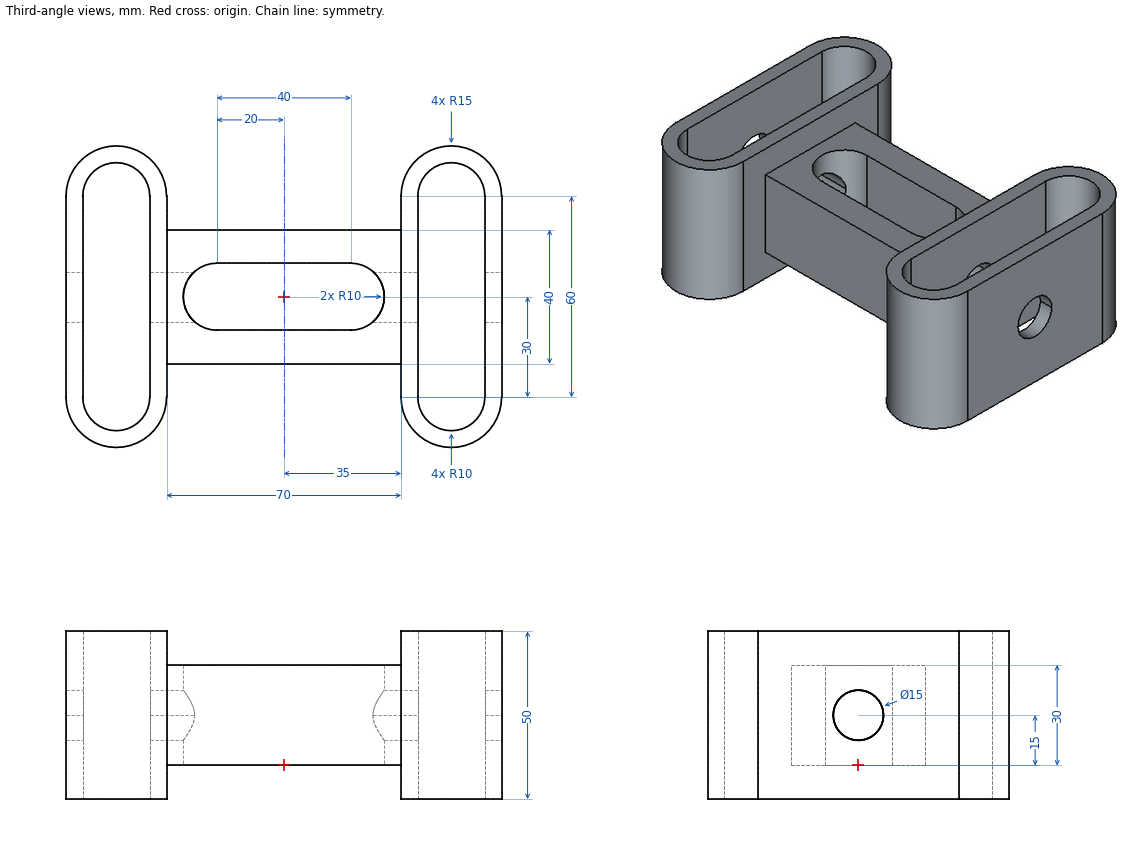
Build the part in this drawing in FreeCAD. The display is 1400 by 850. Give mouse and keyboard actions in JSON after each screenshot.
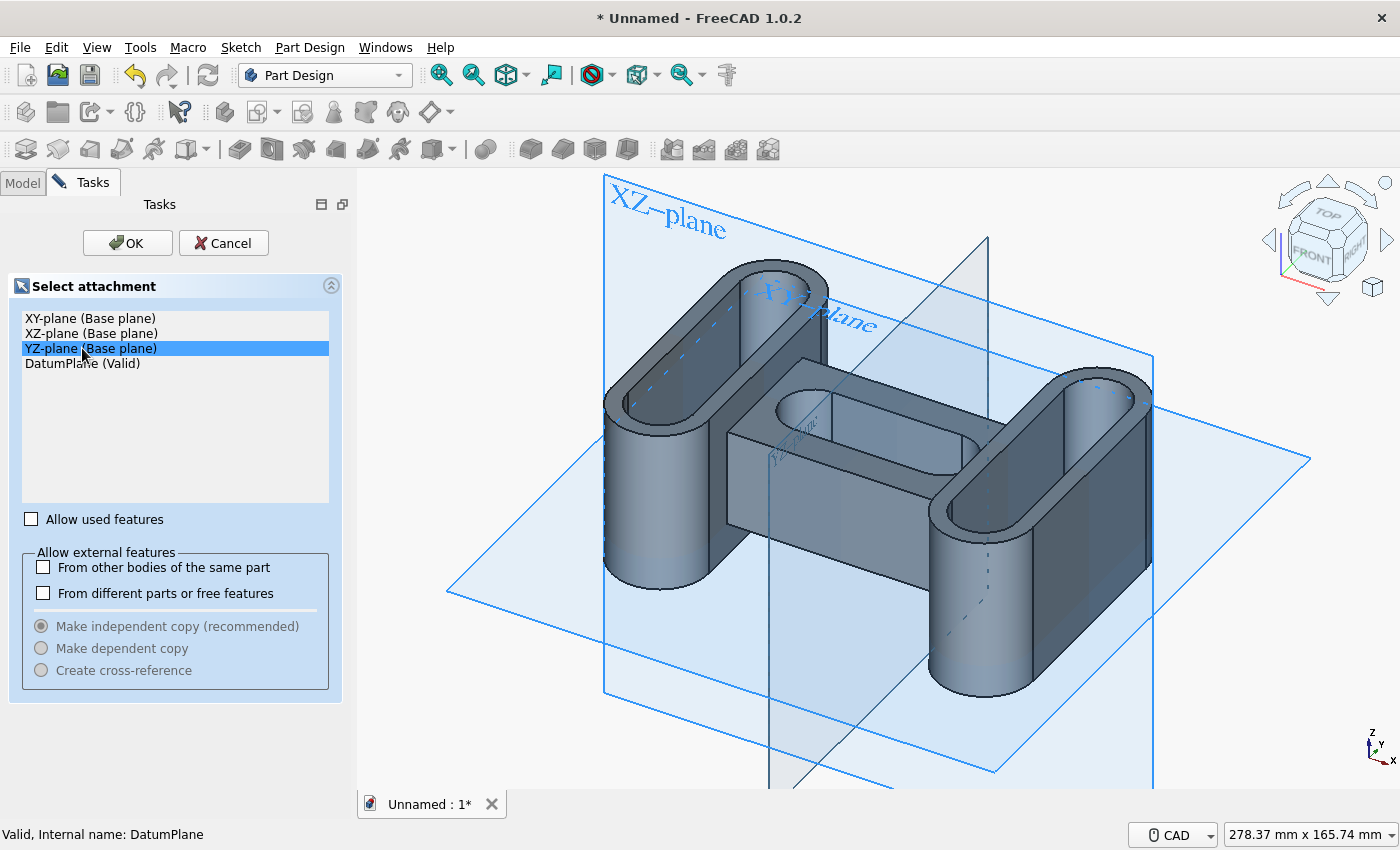
{"action": "left_click", "coordinate": [128, 243]}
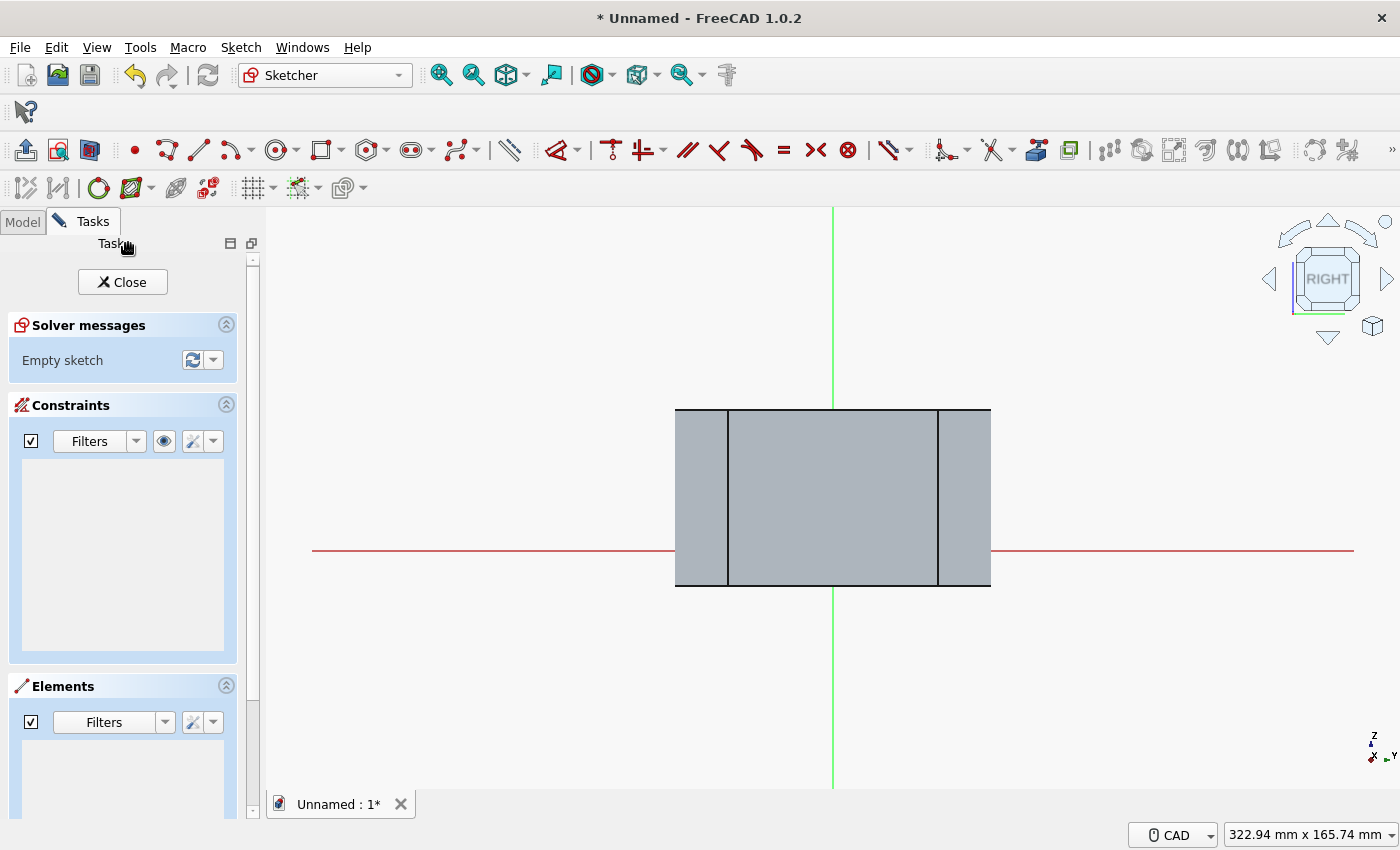
{"action": "key", "text": "q s"}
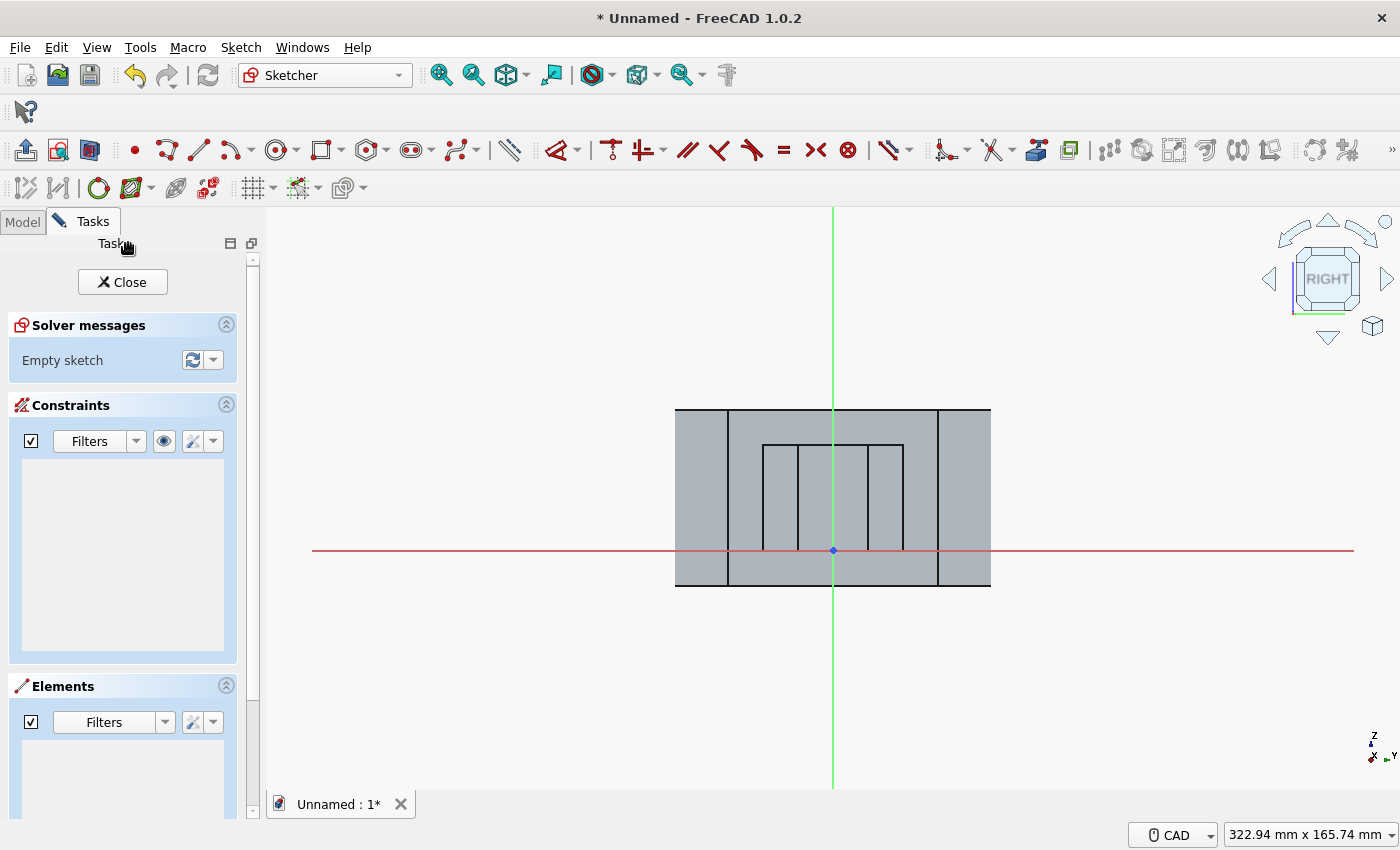
{"action": "scroll", "coordinate": [850, 514], "scroll_direction": "up", "scroll_amount": 8}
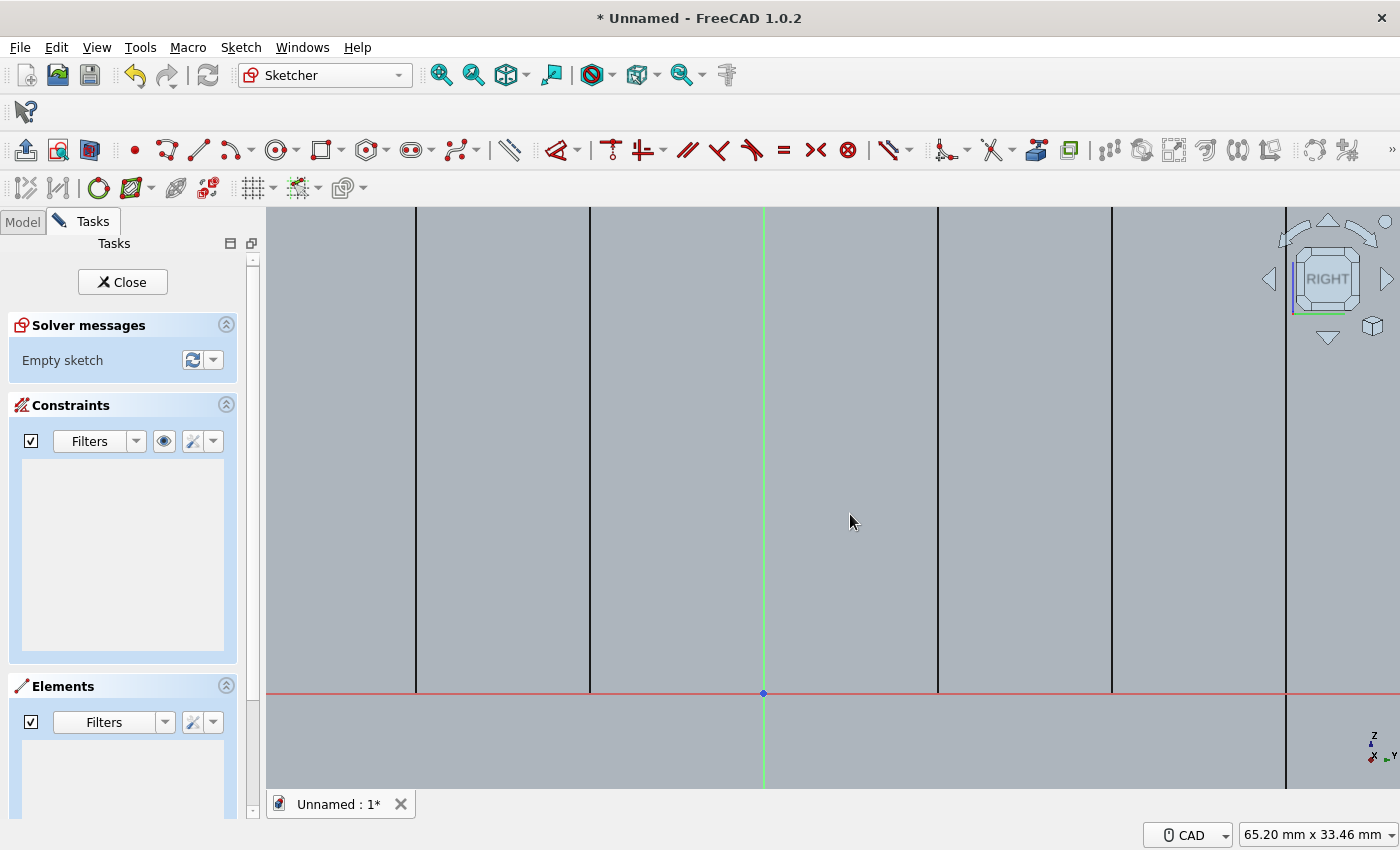
{"action": "left_click", "coordinate": [276, 150]}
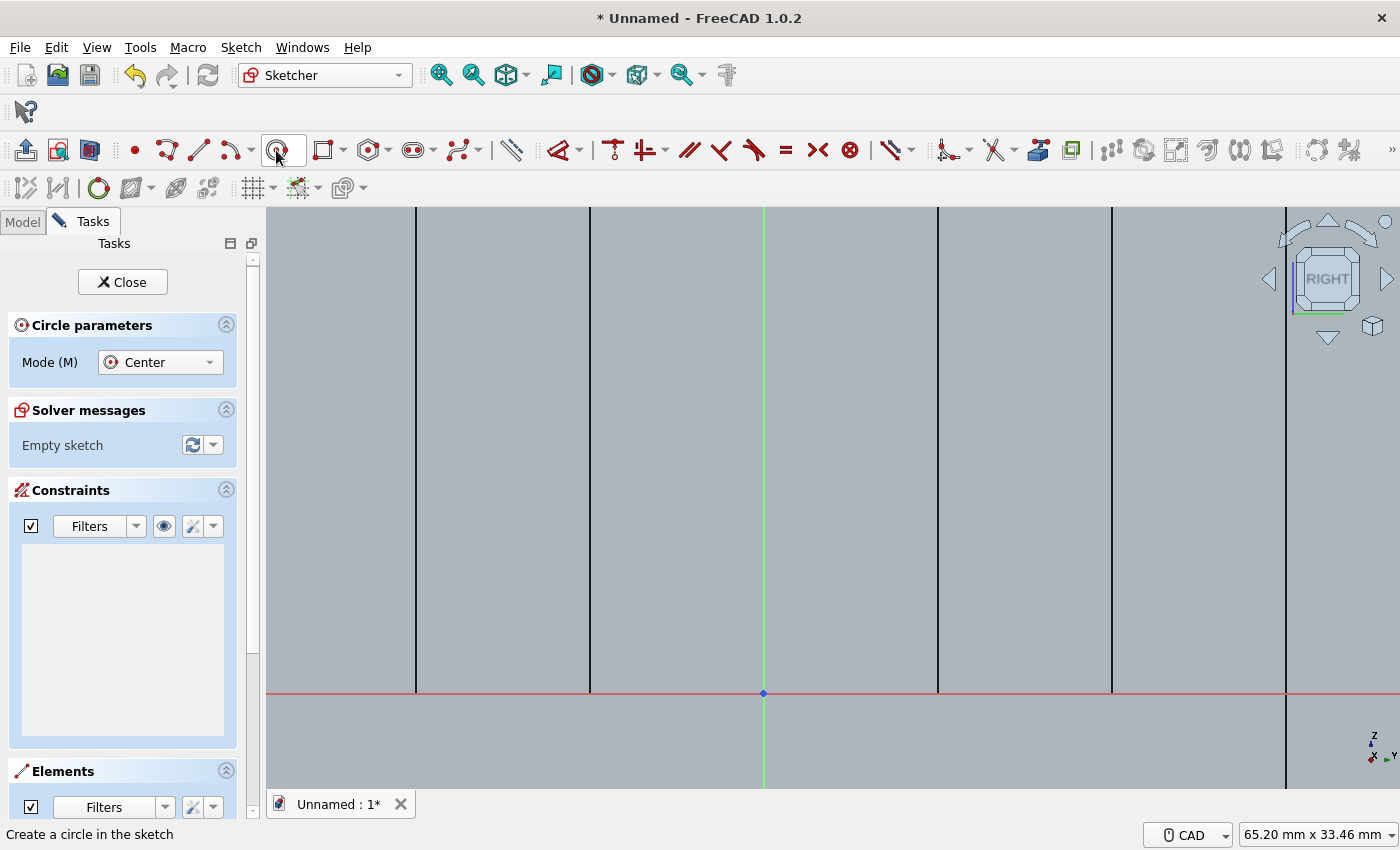
{"action": "left_click", "coordinate": [764, 433]}
{"action": "mouse_move", "coordinate": [856, 340]}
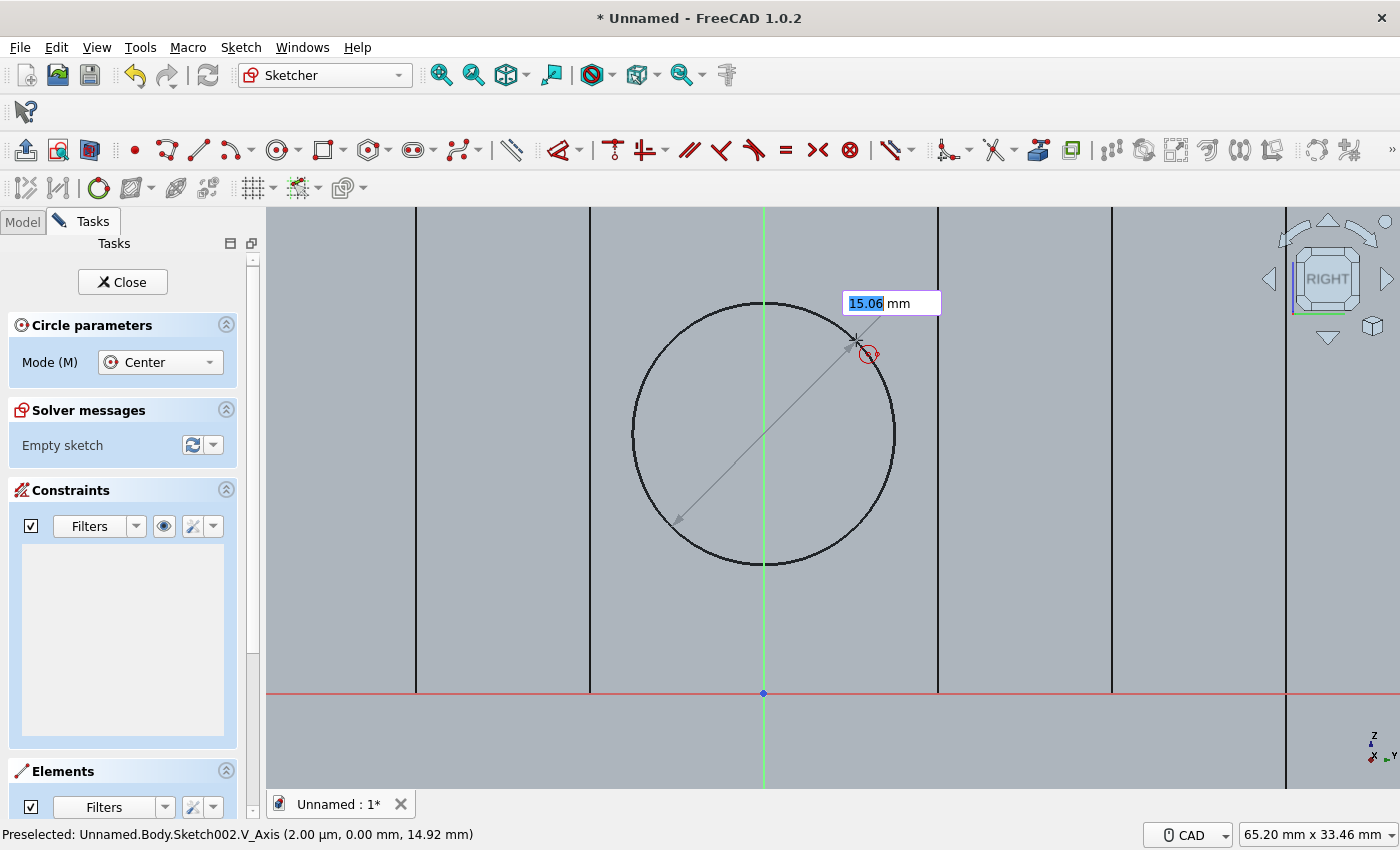
{"action": "type", "text": "15"}
{"action": "key", "text": "Return"}
{"action": "key", "text": "Escape"}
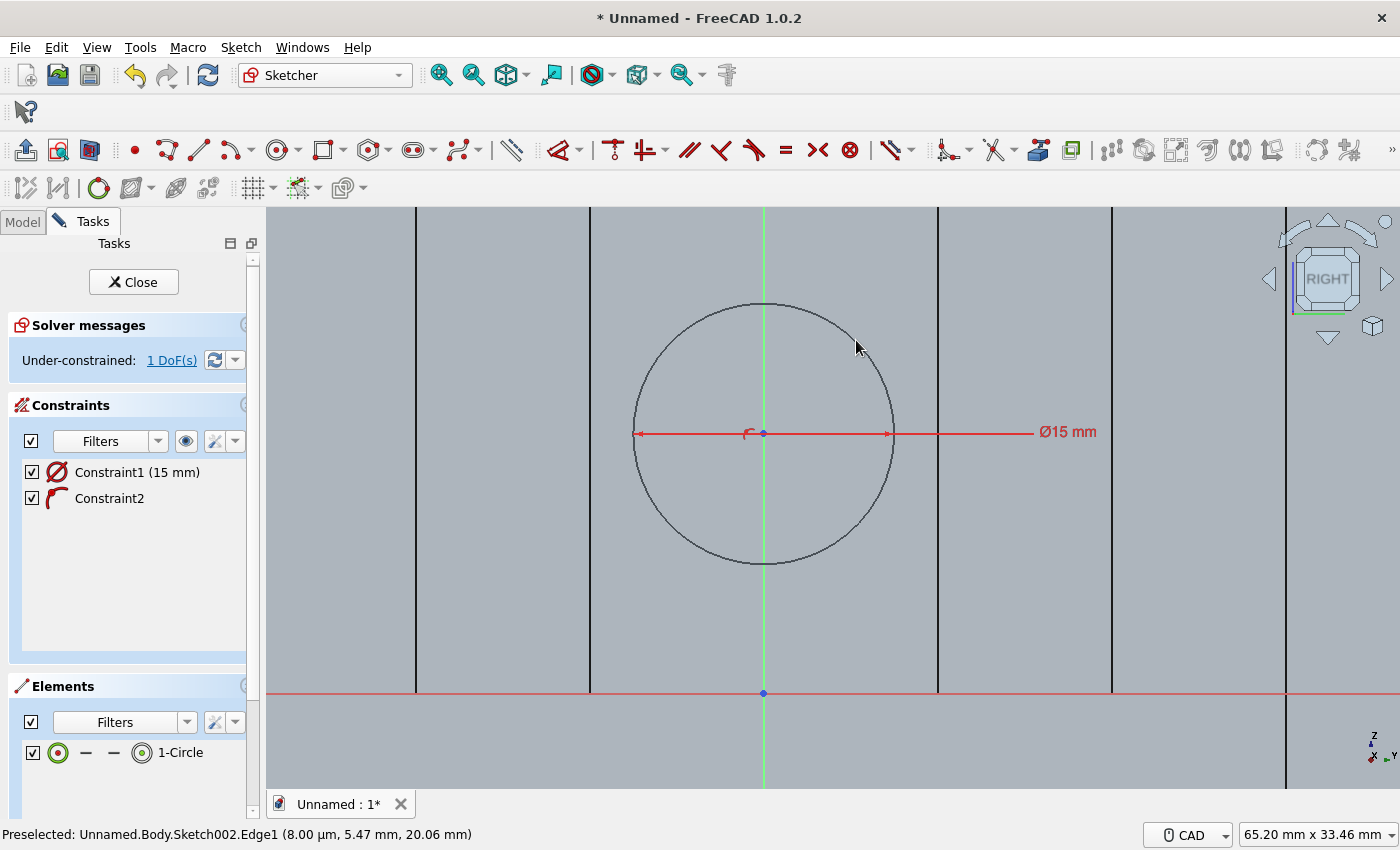
{"action": "key", "text": "d"}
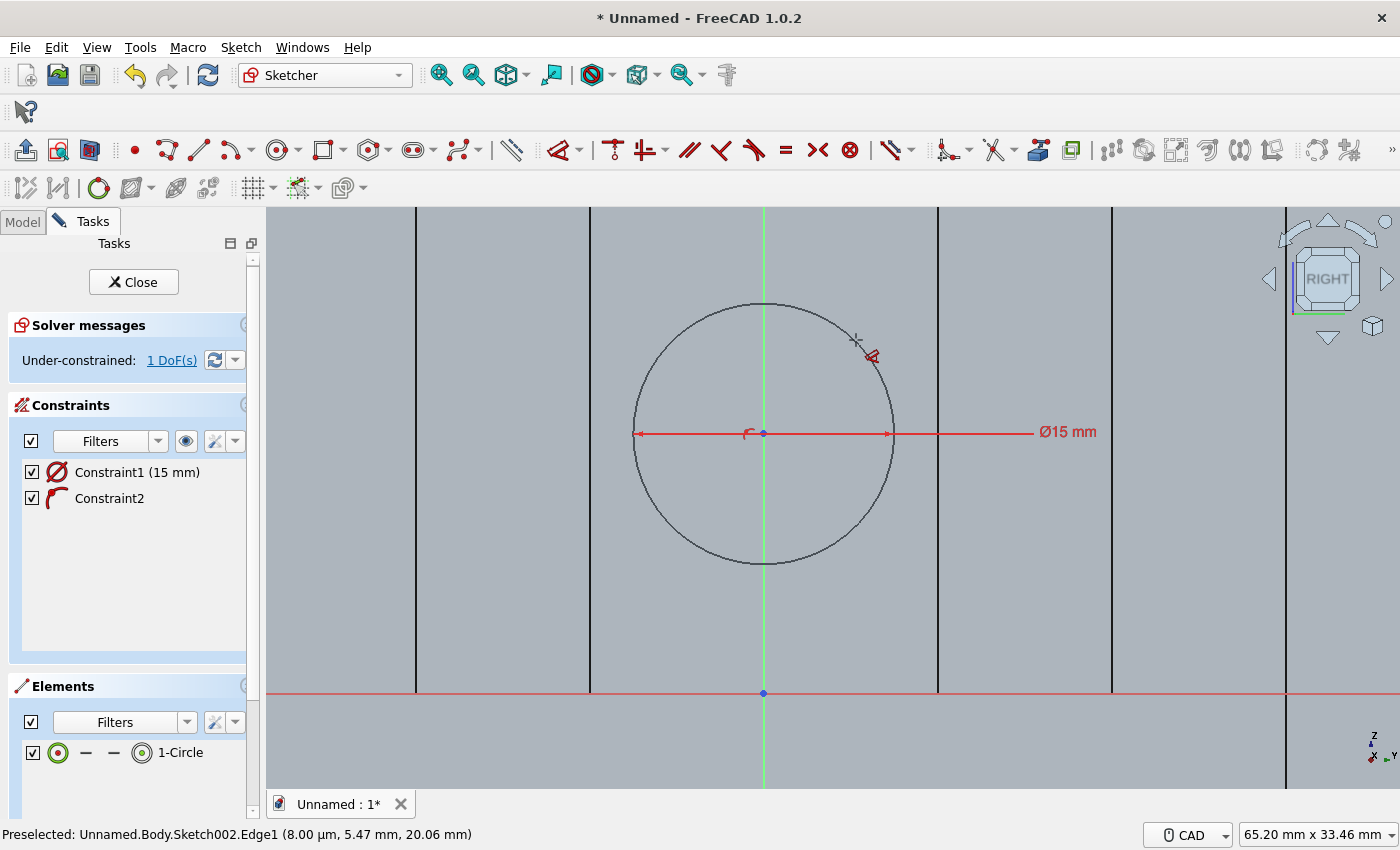
{"action": "left_click", "coordinate": [764, 434]}
{"action": "left_click", "coordinate": [798, 504]}